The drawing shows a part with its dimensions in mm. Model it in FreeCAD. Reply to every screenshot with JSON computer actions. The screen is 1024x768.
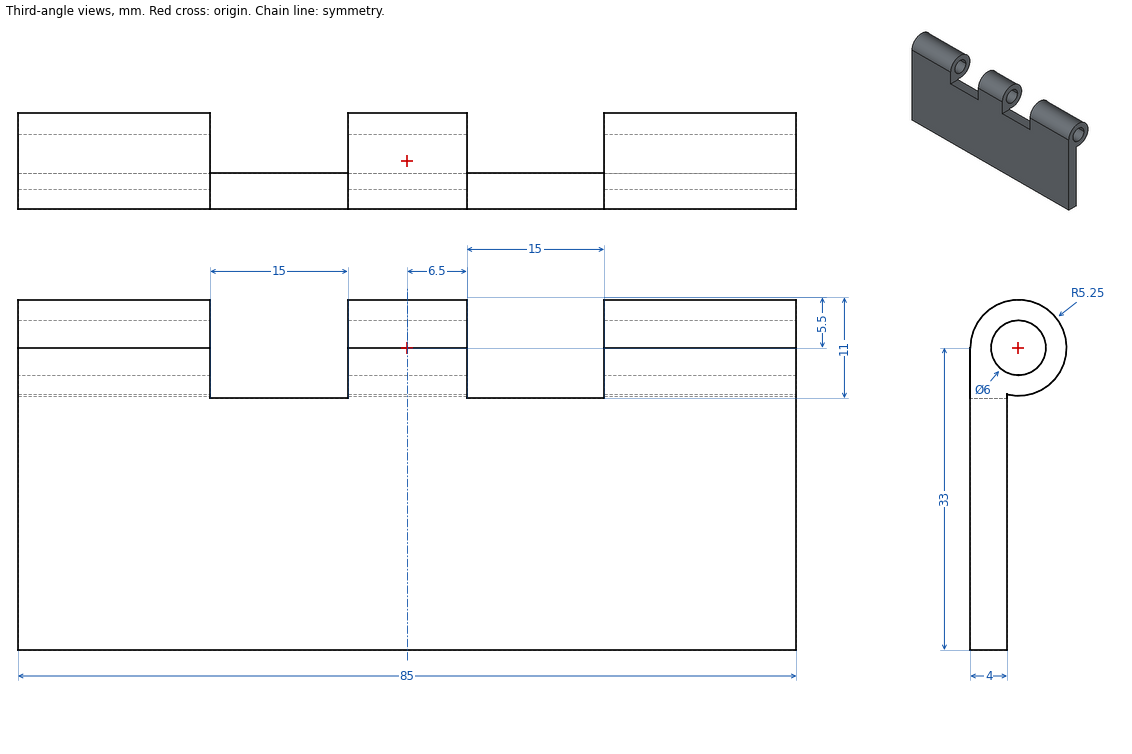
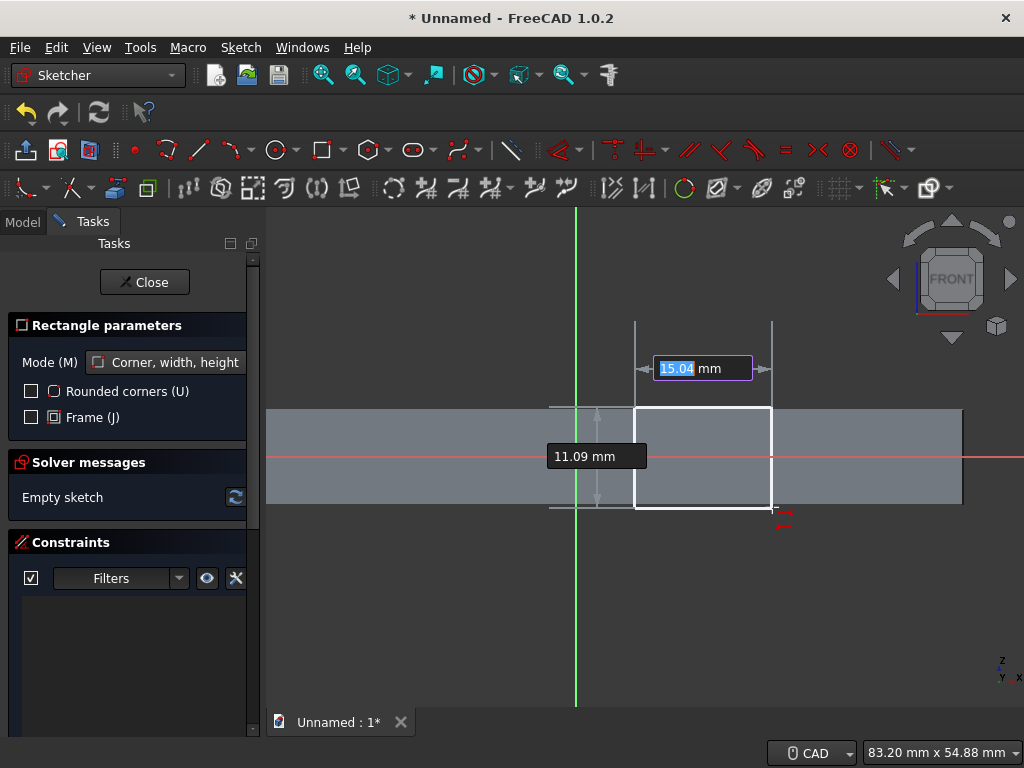
{"action": "type", "text": "15"}
{"action": "key", "text": "Tab"}
{"action": "type", "text": "11"}
{"action": "key", "text": "Return"}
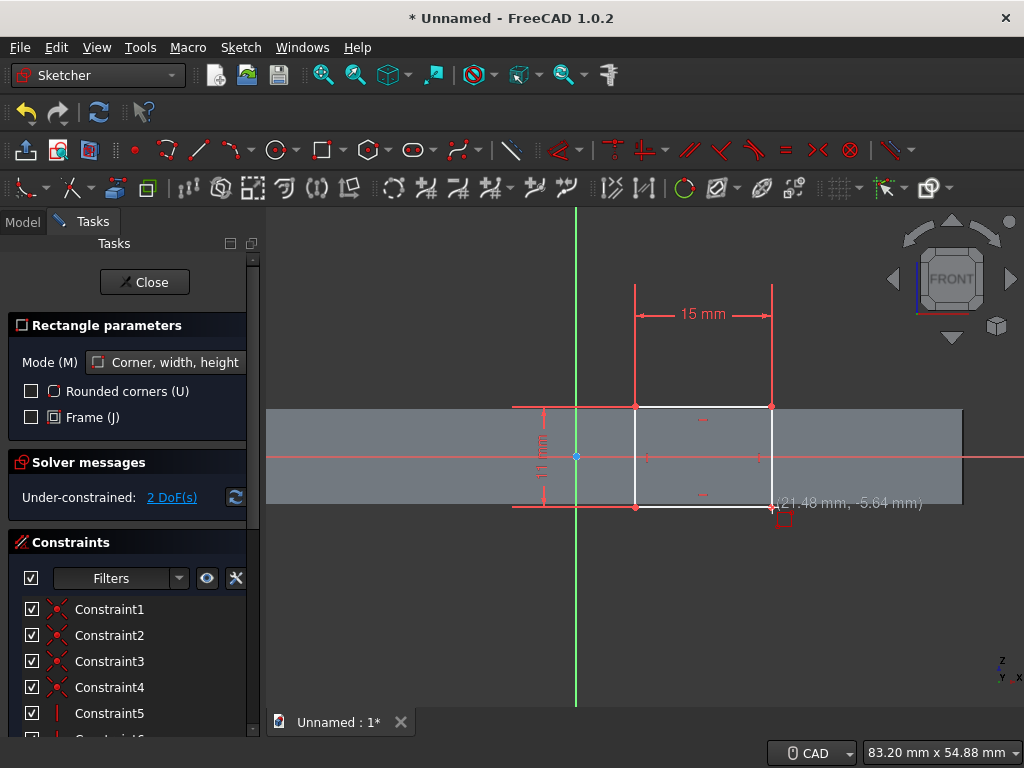
{"action": "left_click", "coordinate": [380, 406]}
{"action": "mouse_move", "coordinate": [517, 507]}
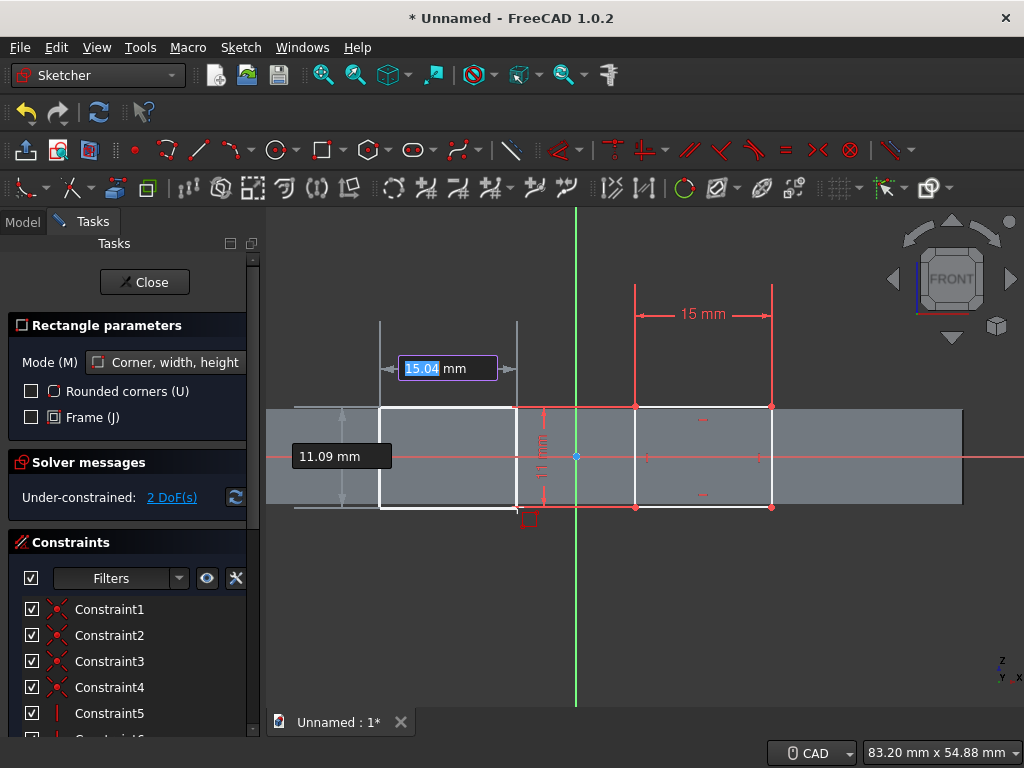
{"action": "type", "text": "15"}
{"action": "key", "text": "Tab"}
{"action": "type", "text": "11"}
{"action": "key", "text": "Return"}
{"action": "key", "text": "Escape"}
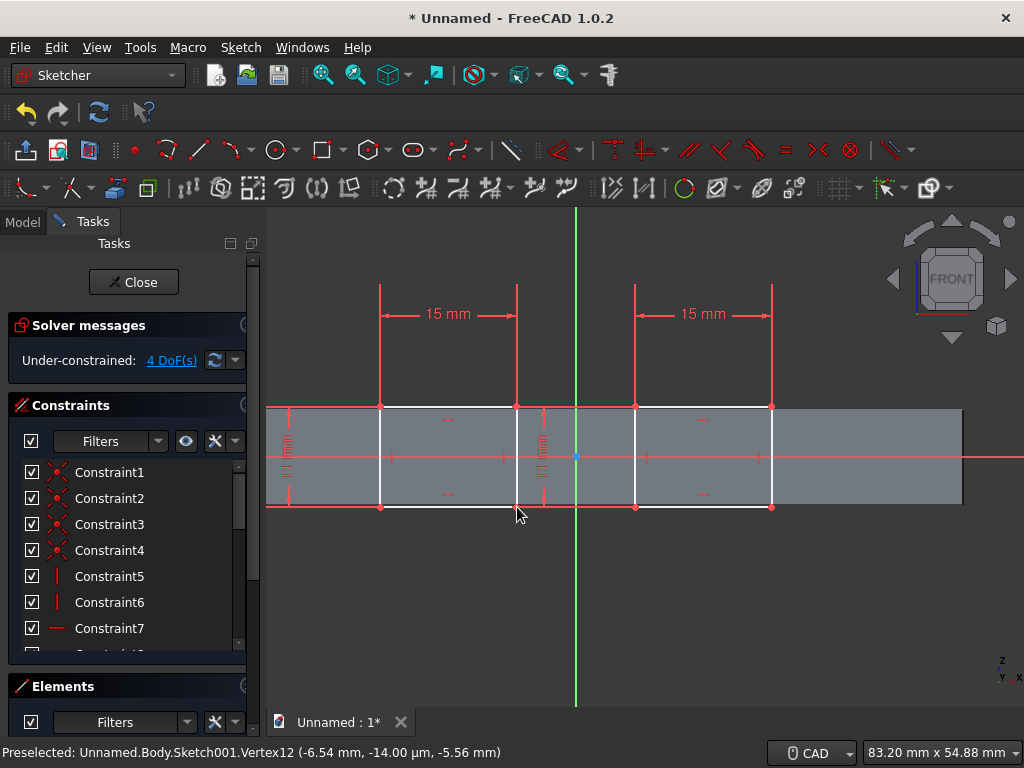
{"action": "left_click", "coordinate": [772, 407]}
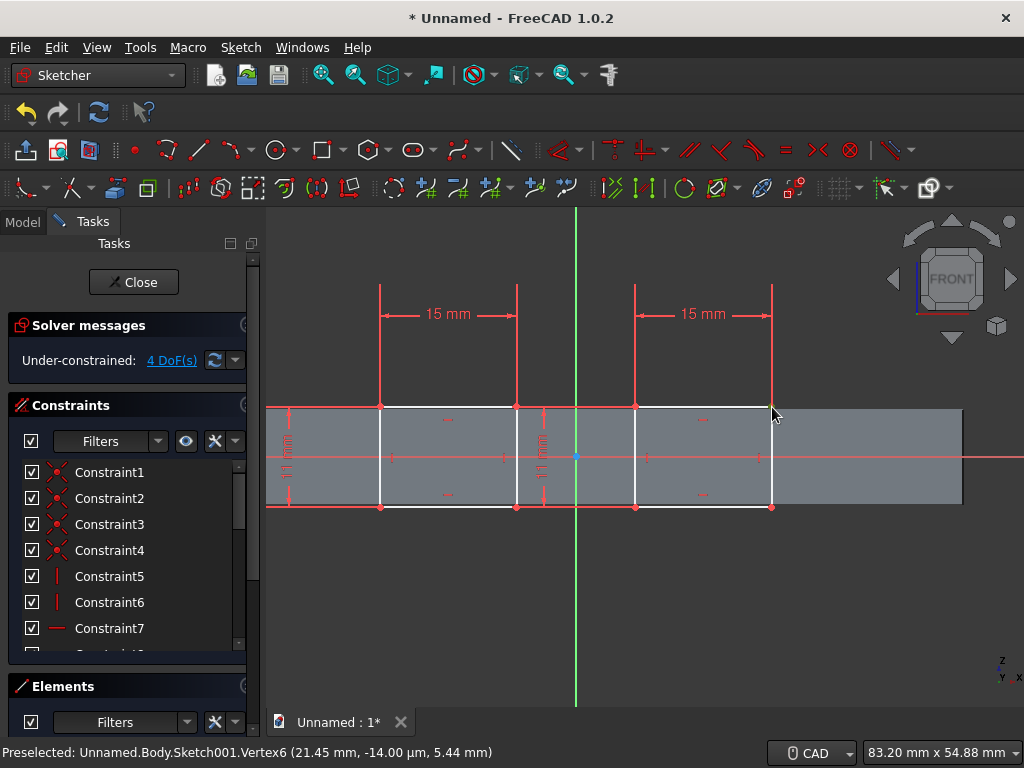
{"action": "left_click", "coordinate": [380, 407]}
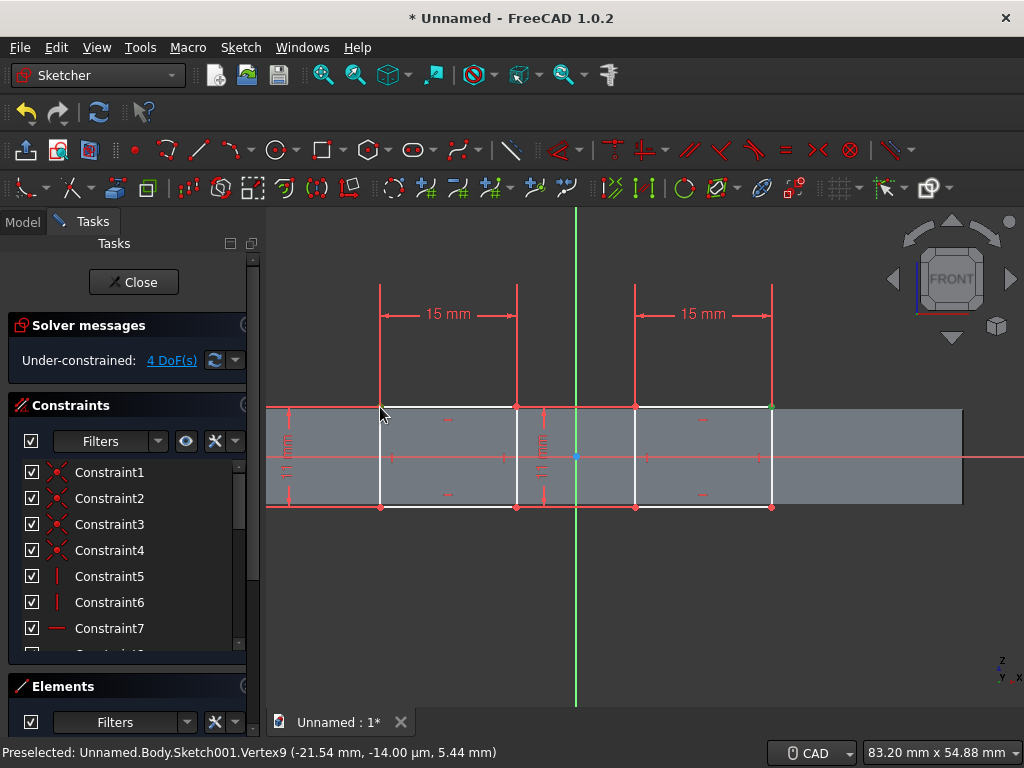
{"action": "left_click", "coordinate": [576, 647]}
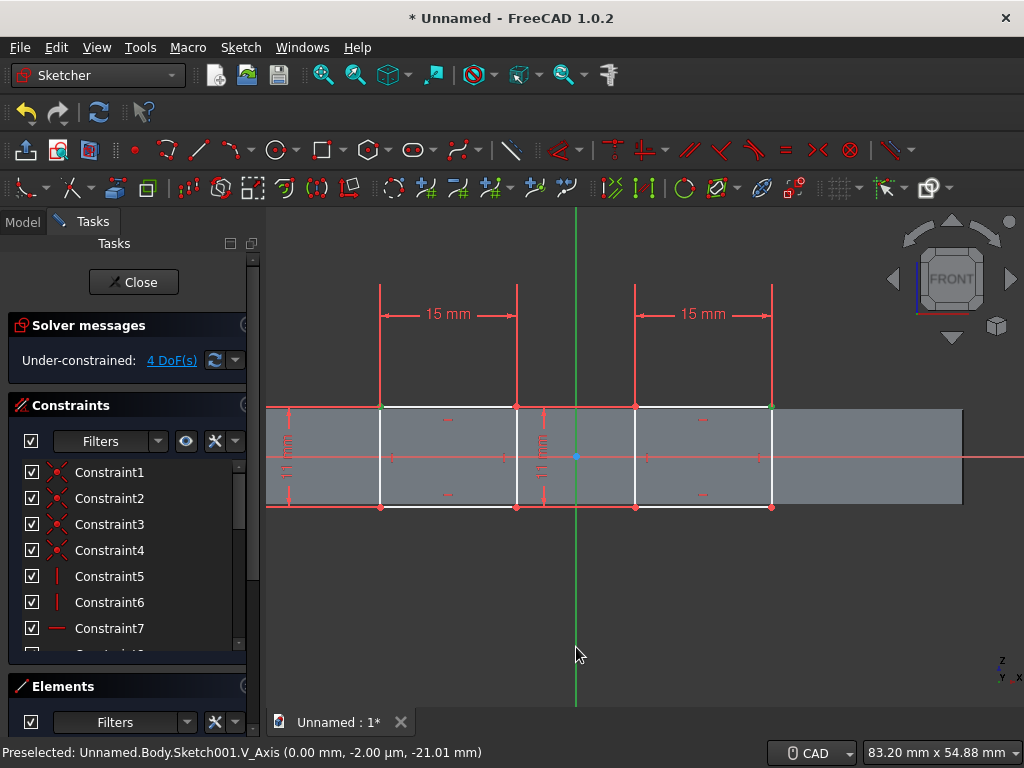
{"action": "left_click", "coordinate": [818, 150]}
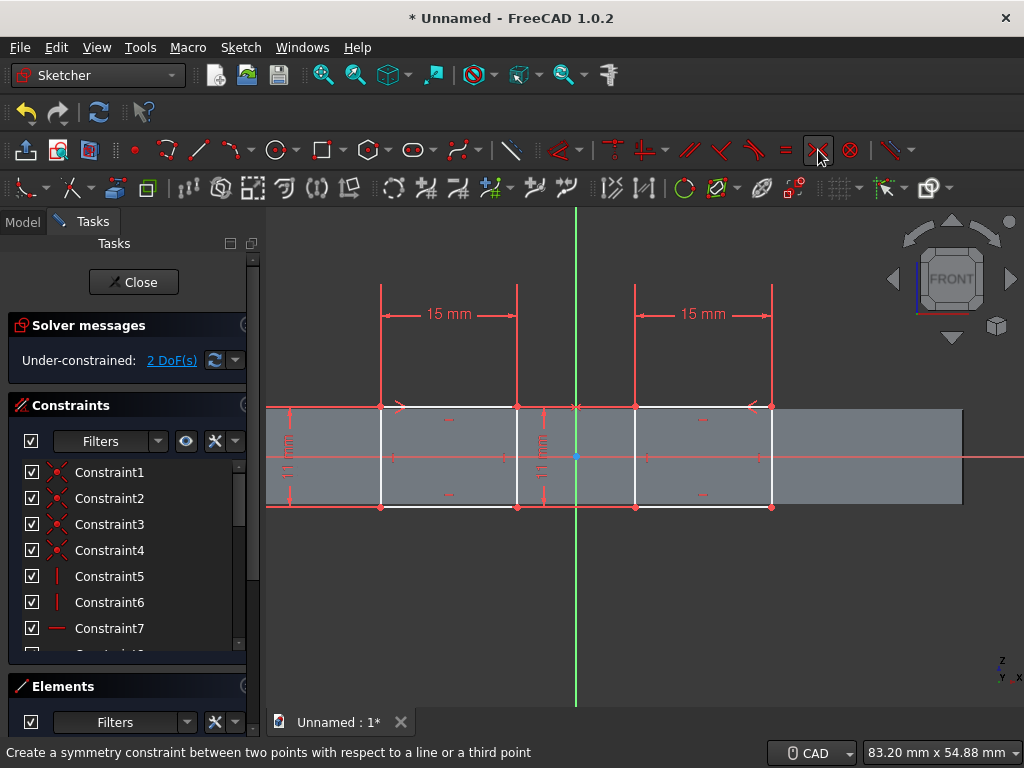
{"action": "left_click", "coordinate": [558, 150]}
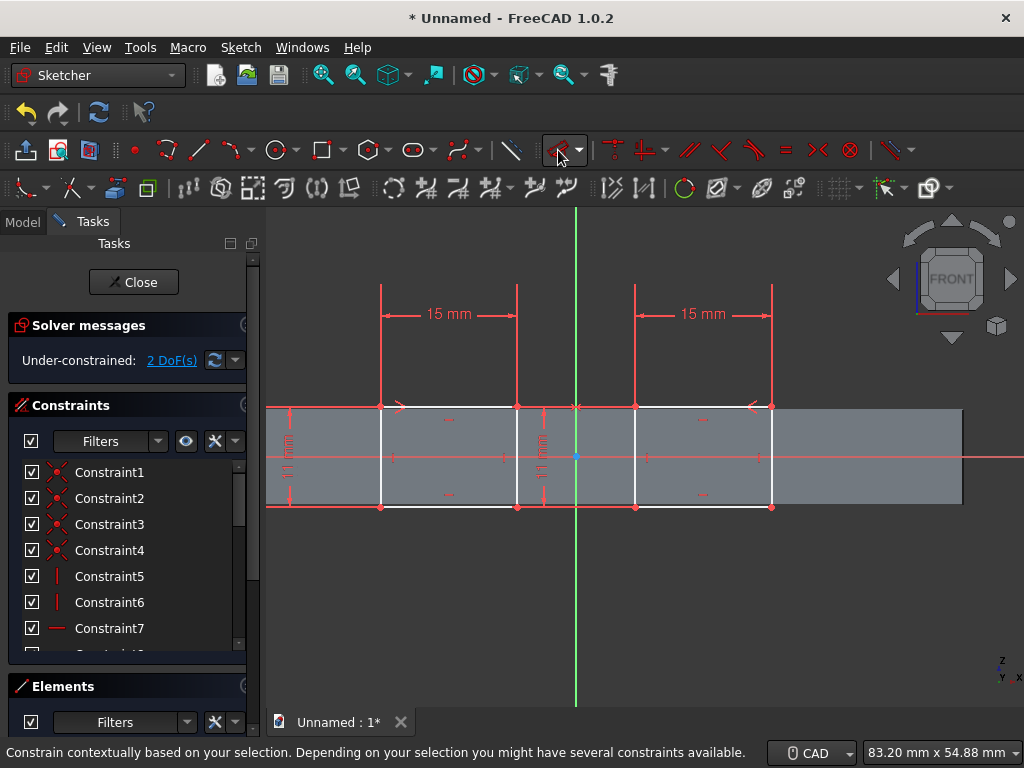
{"action": "left_click", "coordinate": [635, 407]}
{"action": "left_click", "coordinate": [606, 373]}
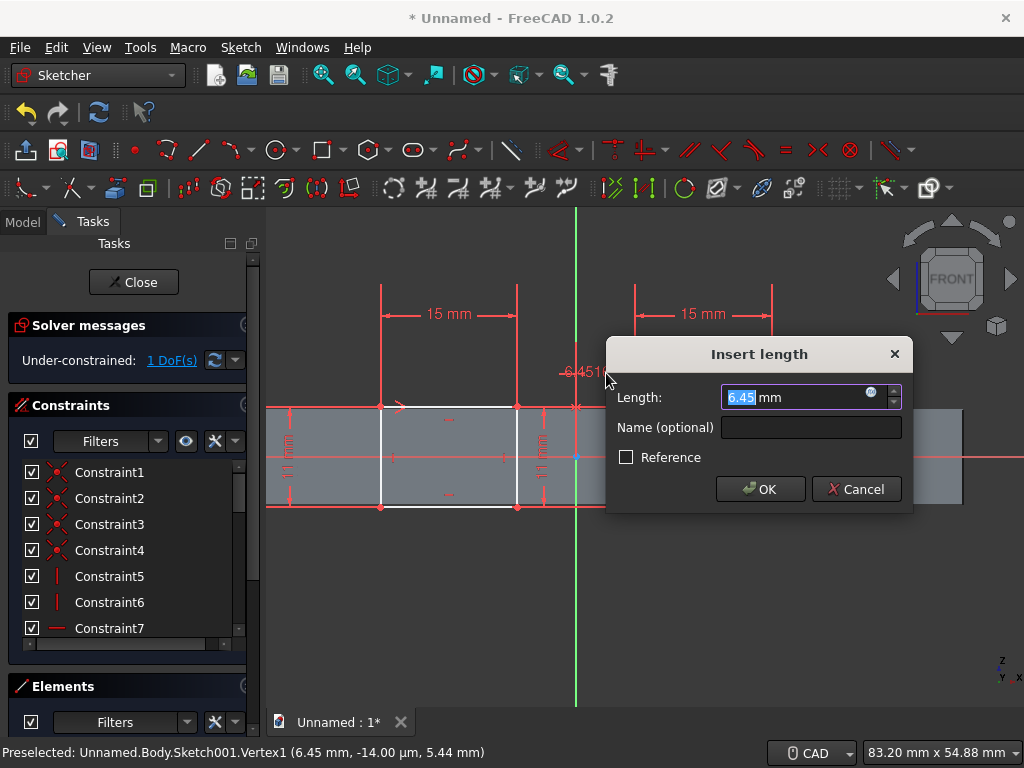
{"action": "type", "text": "6.5"}
{"action": "key", "text": "Return"}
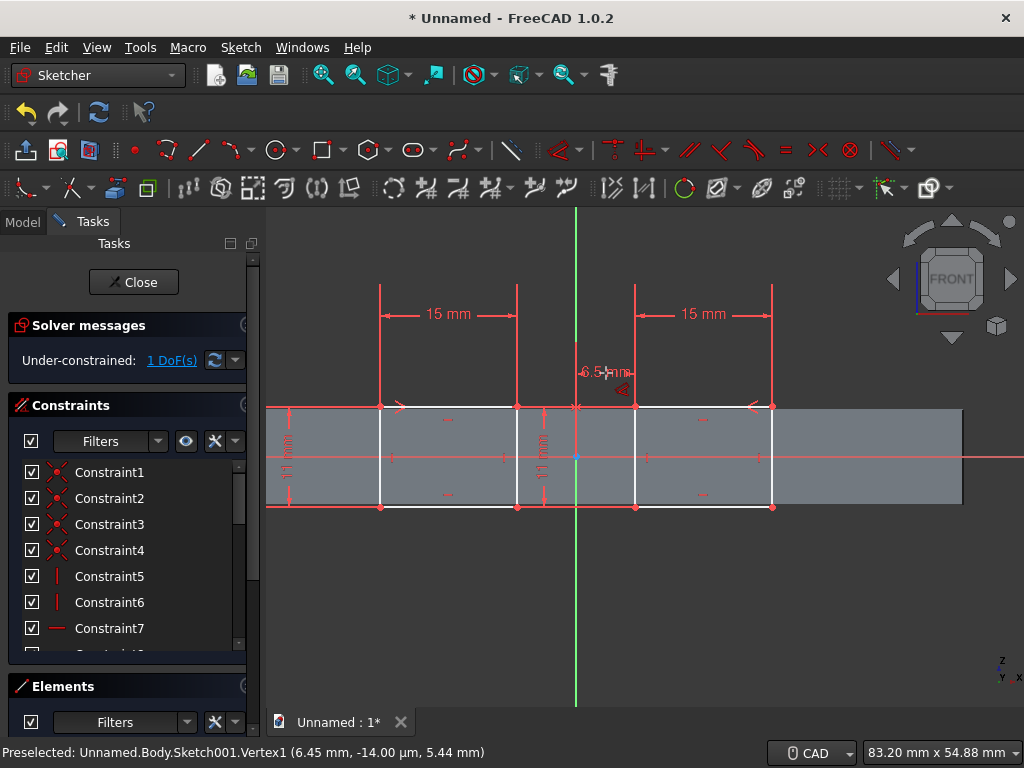
{"action": "left_click", "coordinate": [635, 407]}
{"action": "left_click", "coordinate": [669, 432]}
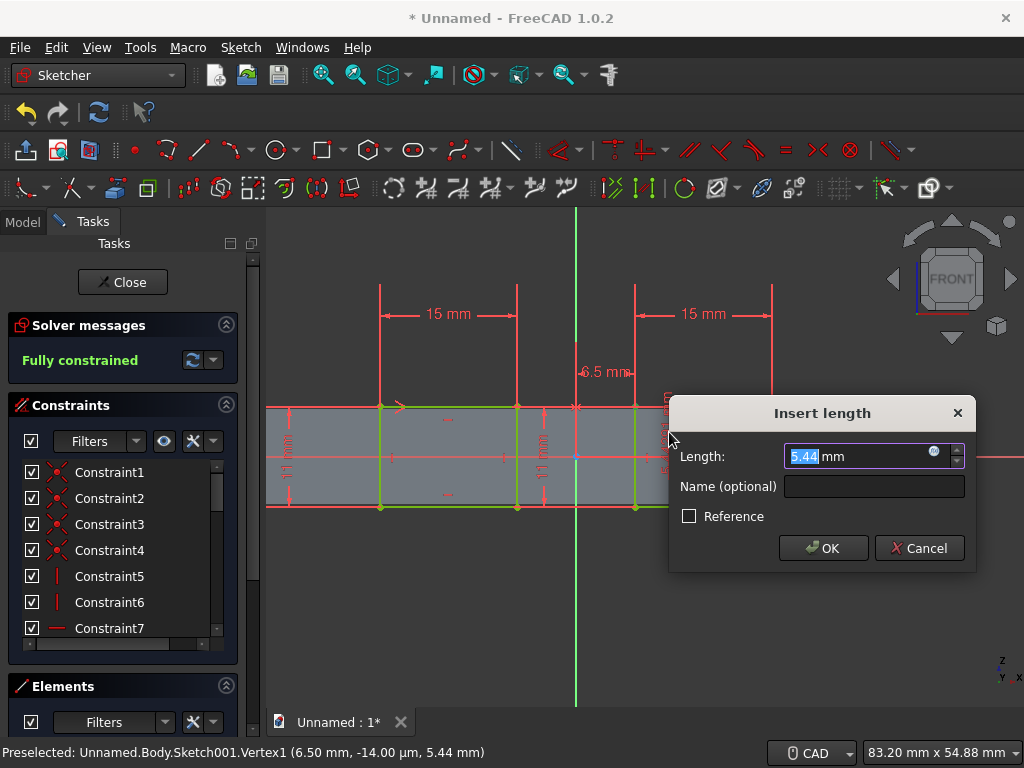
{"action": "type", "text": "5.5"}
{"action": "key", "text": "Return"}
{"action": "key", "text": "Escape"}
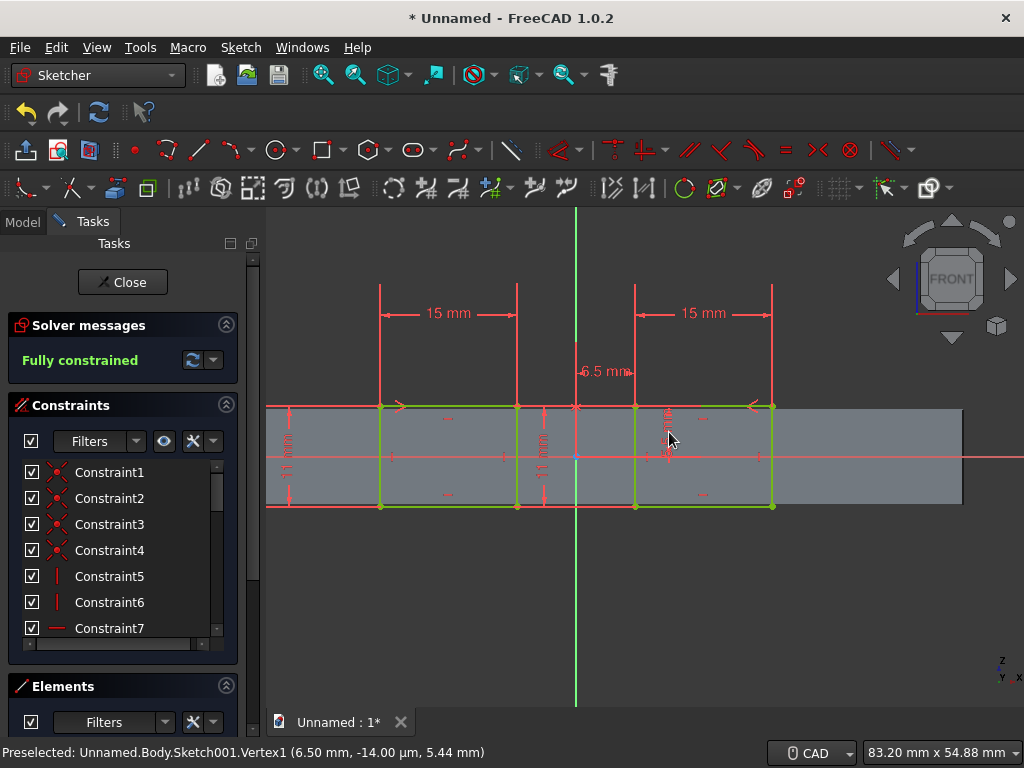
{"action": "left_click", "coordinate": [123, 282]}